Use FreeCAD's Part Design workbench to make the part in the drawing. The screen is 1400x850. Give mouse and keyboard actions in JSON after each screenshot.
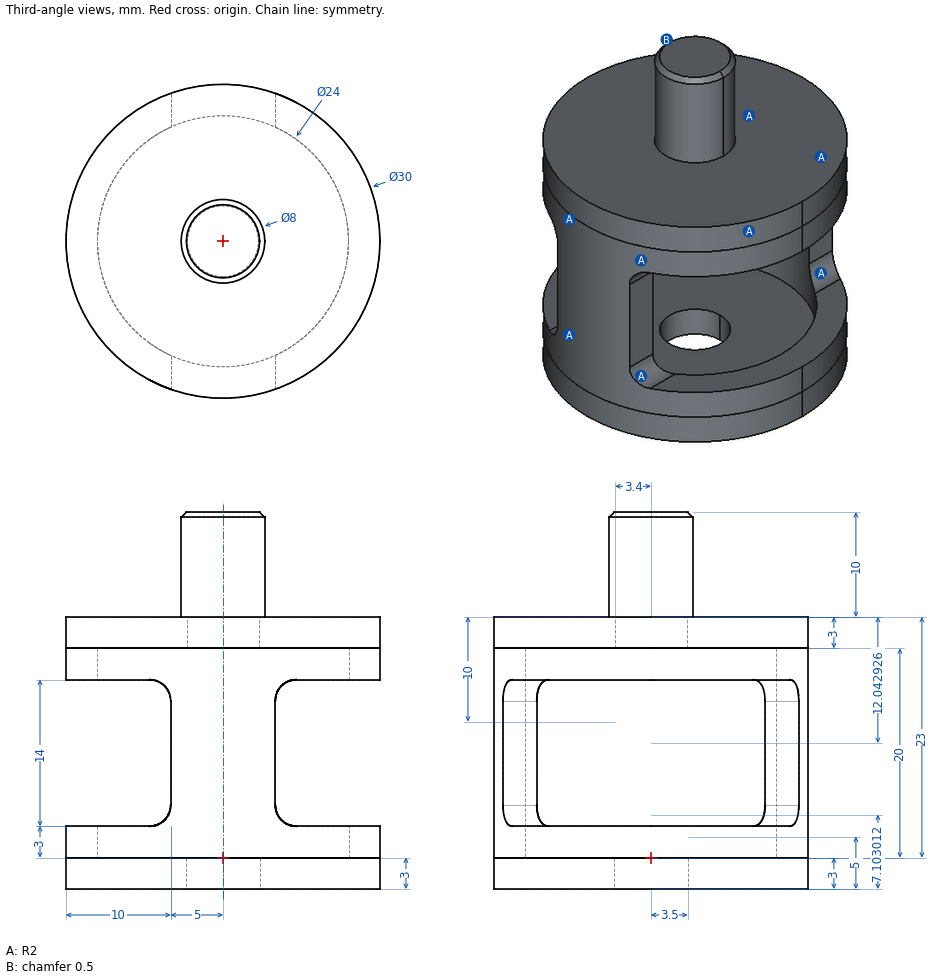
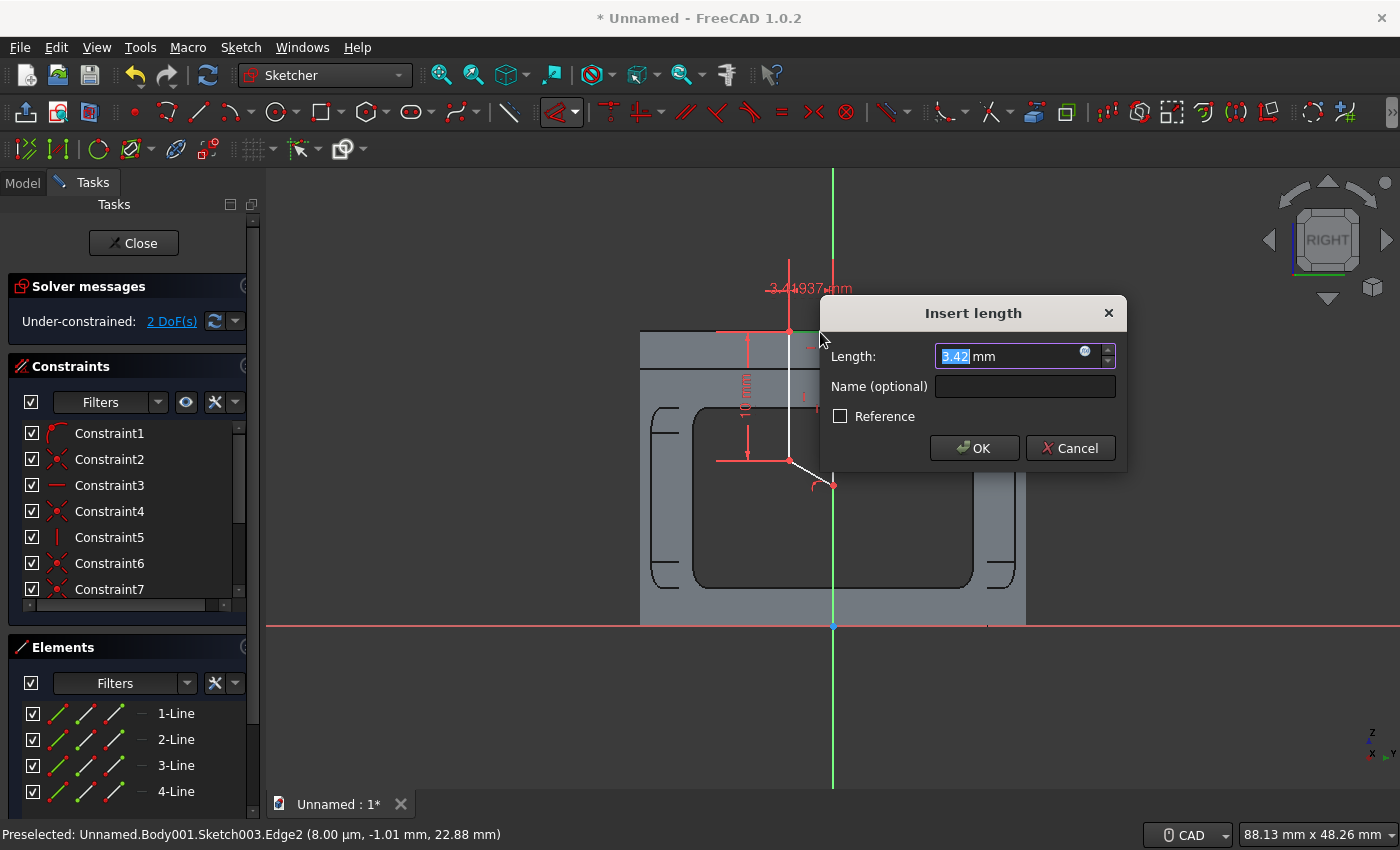
{"action": "type", "text": "3.4"}
{"action": "key", "text": "Return"}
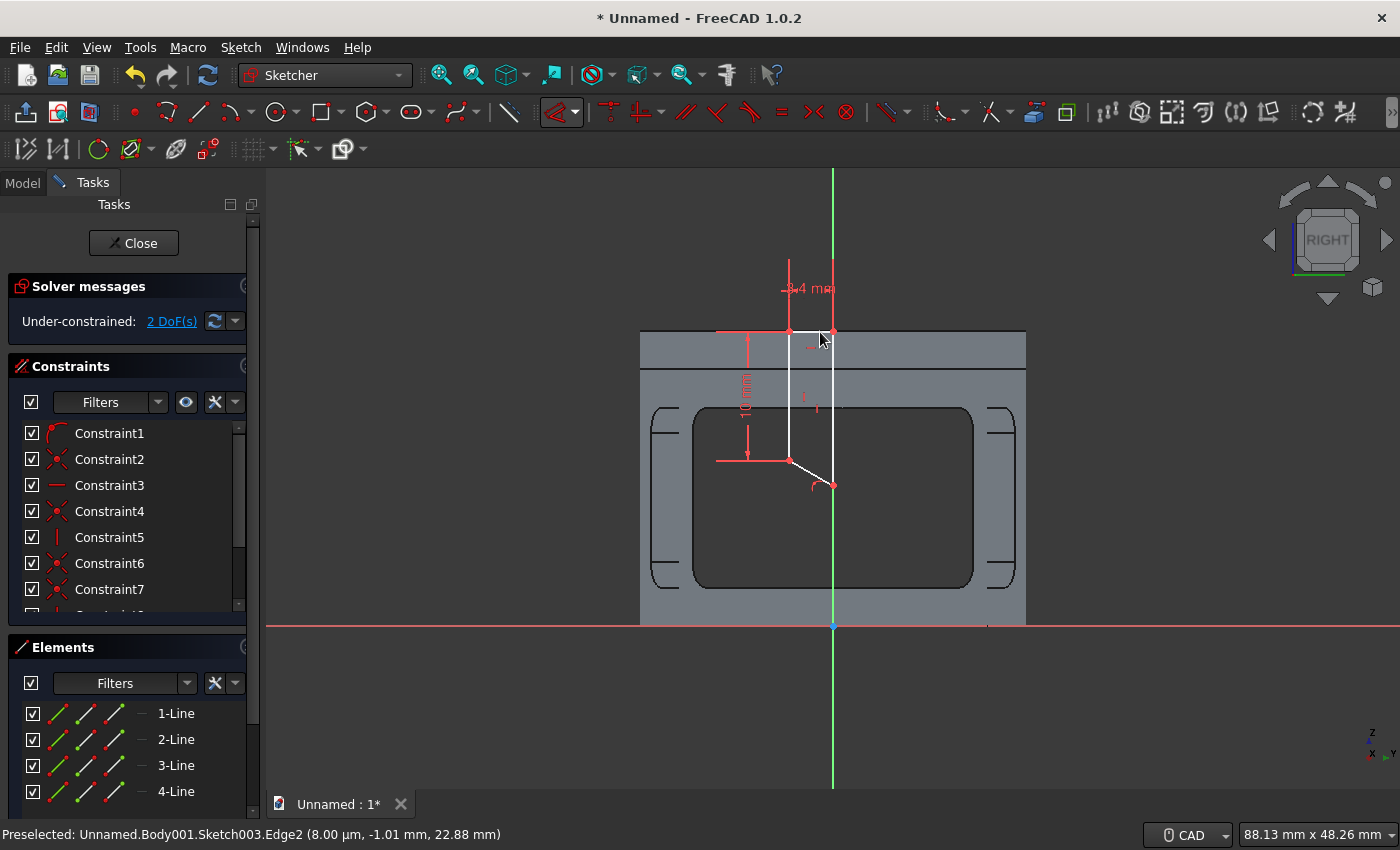
{"action": "left_click", "coordinate": [833, 332]}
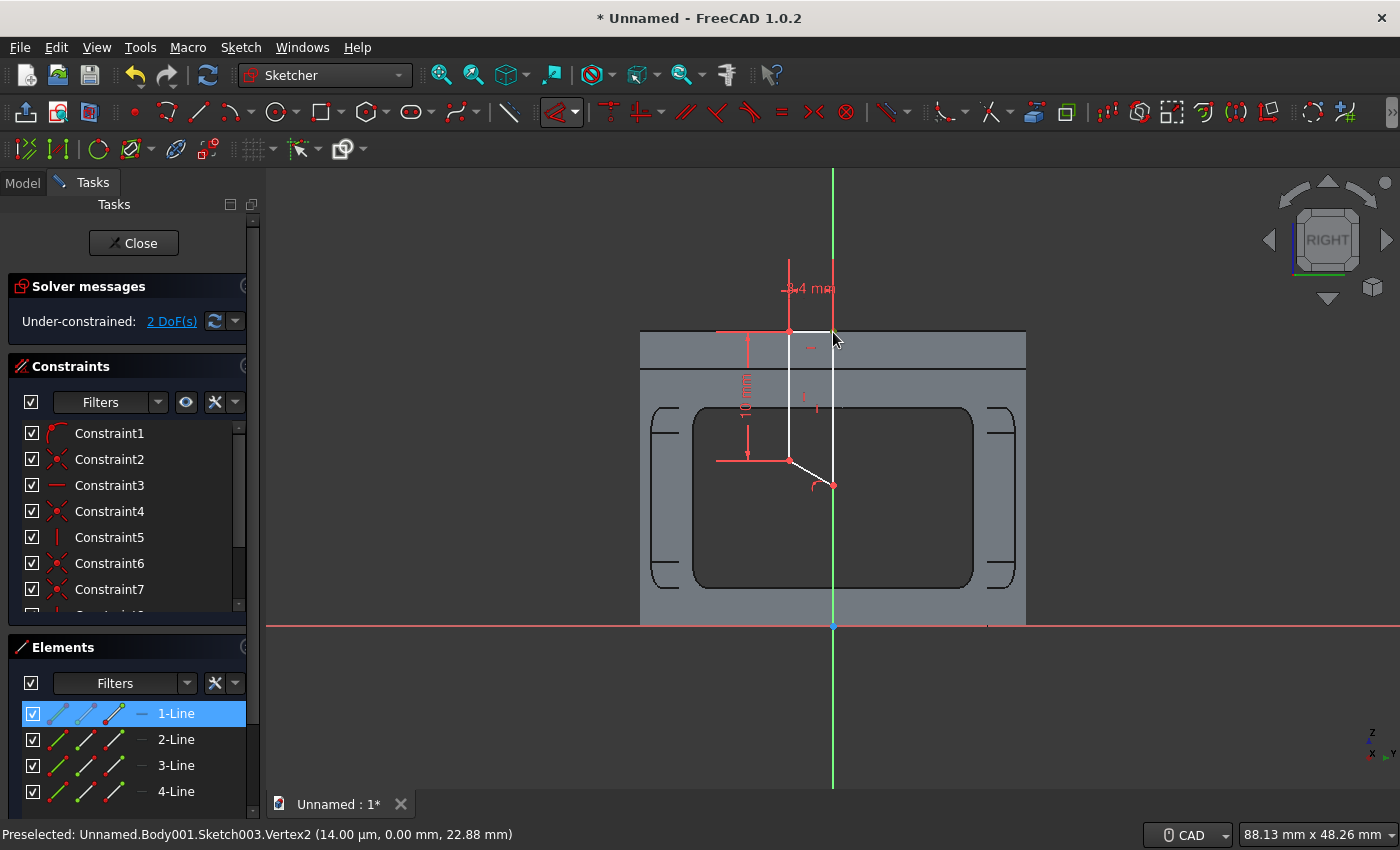
{"action": "key", "text": "i"}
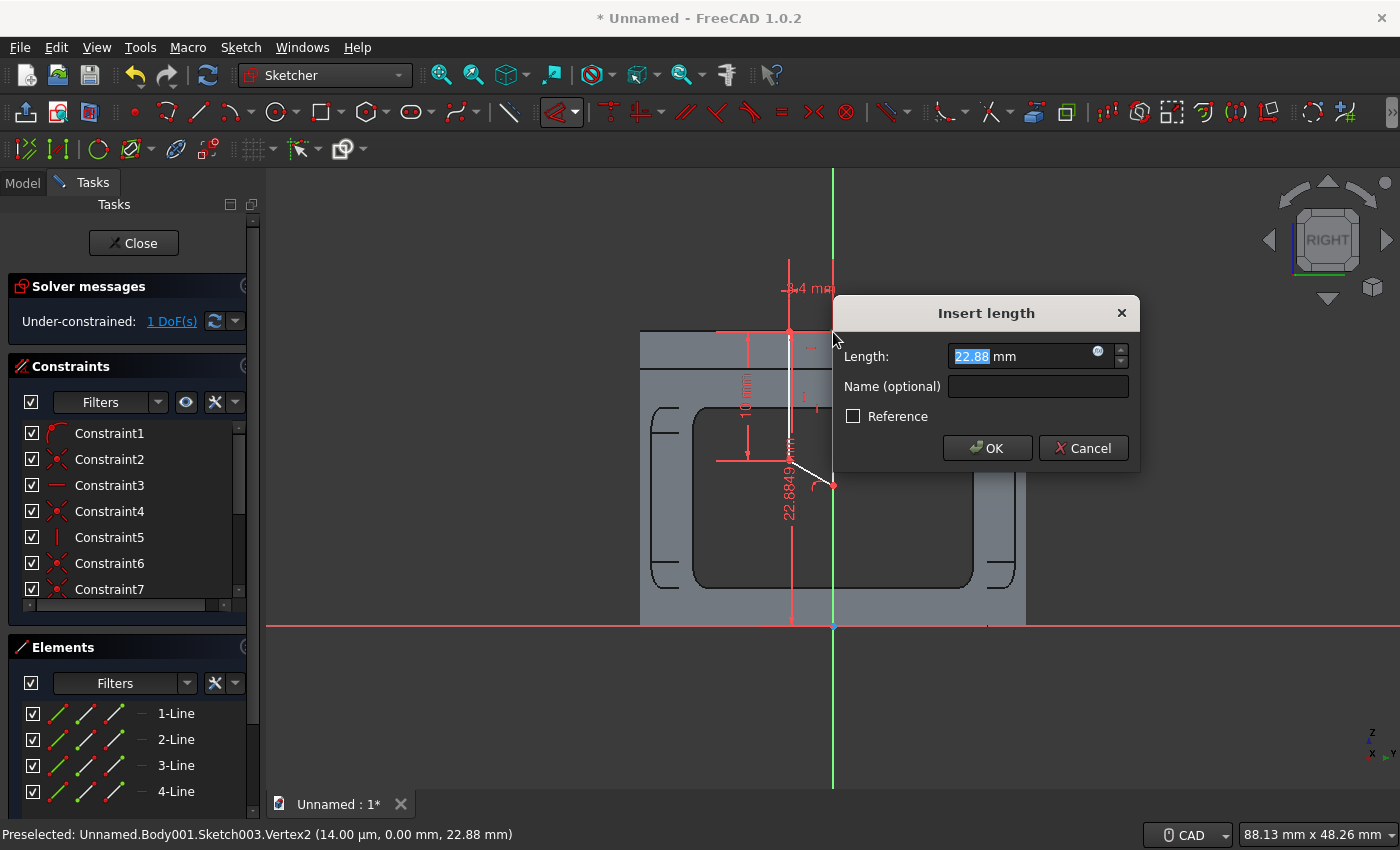
{"action": "type", "text": "23"}
{"action": "key", "text": "Return"}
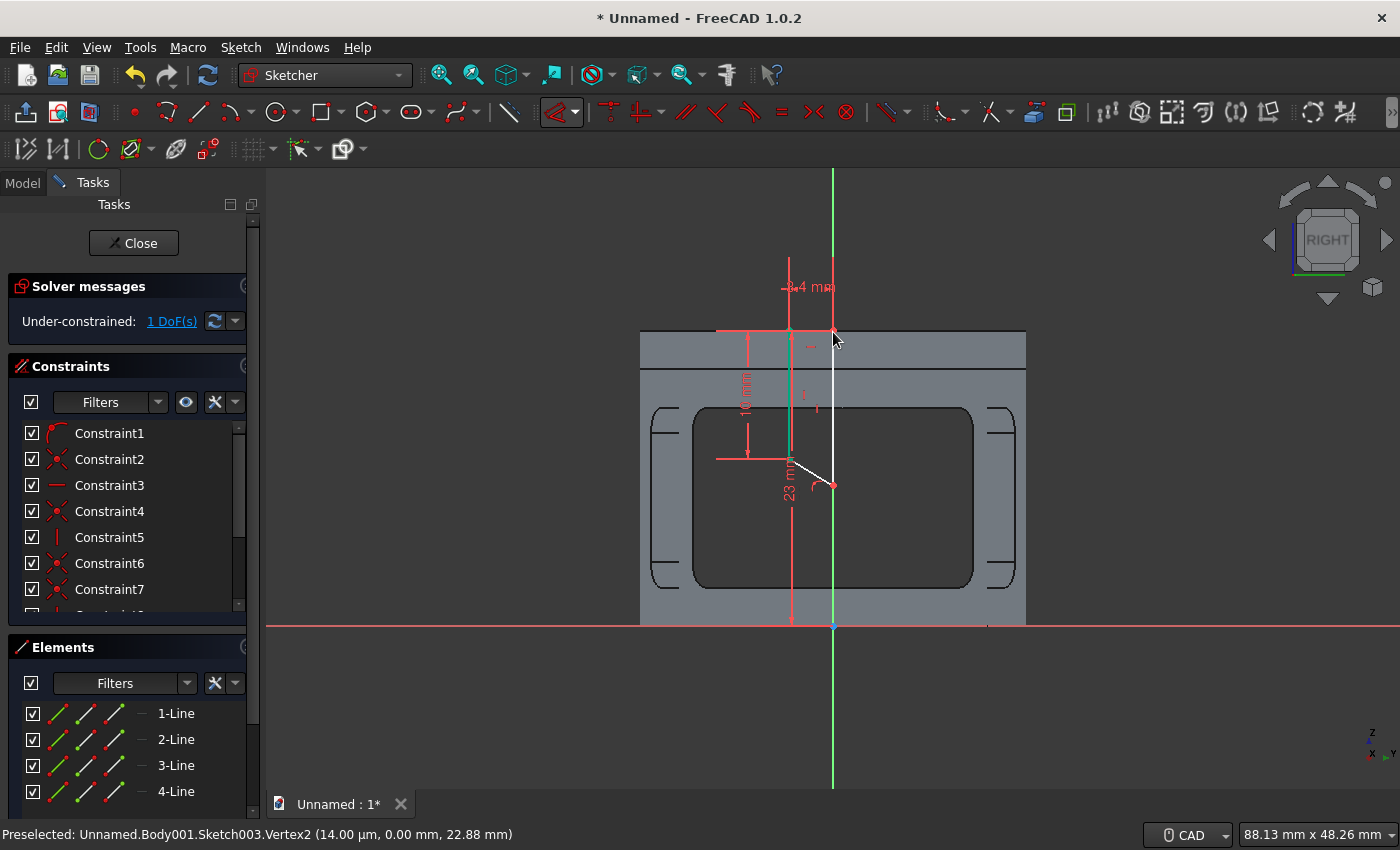
{"action": "left_click", "coordinate": [833, 439]}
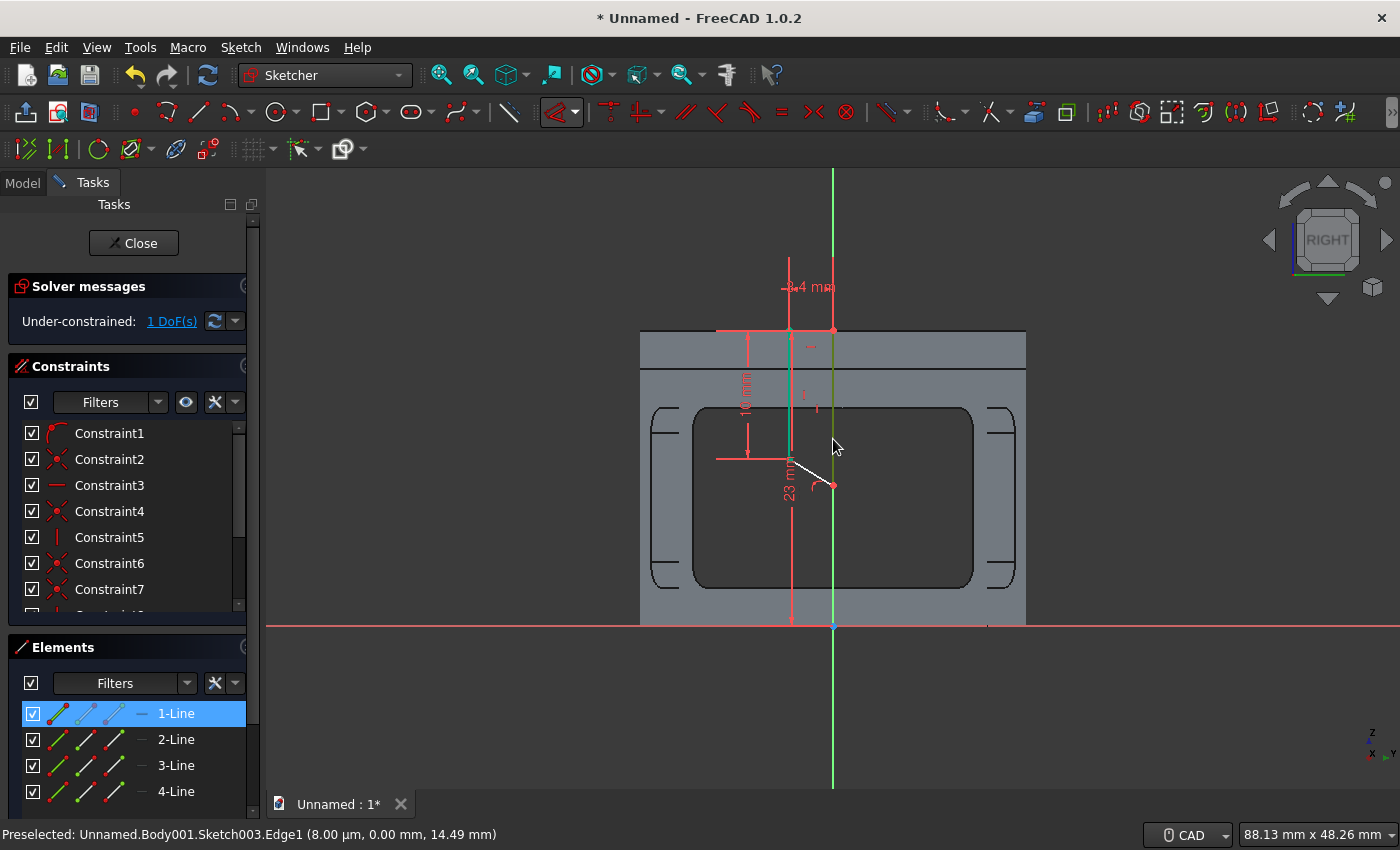
{"action": "key", "text": "i"}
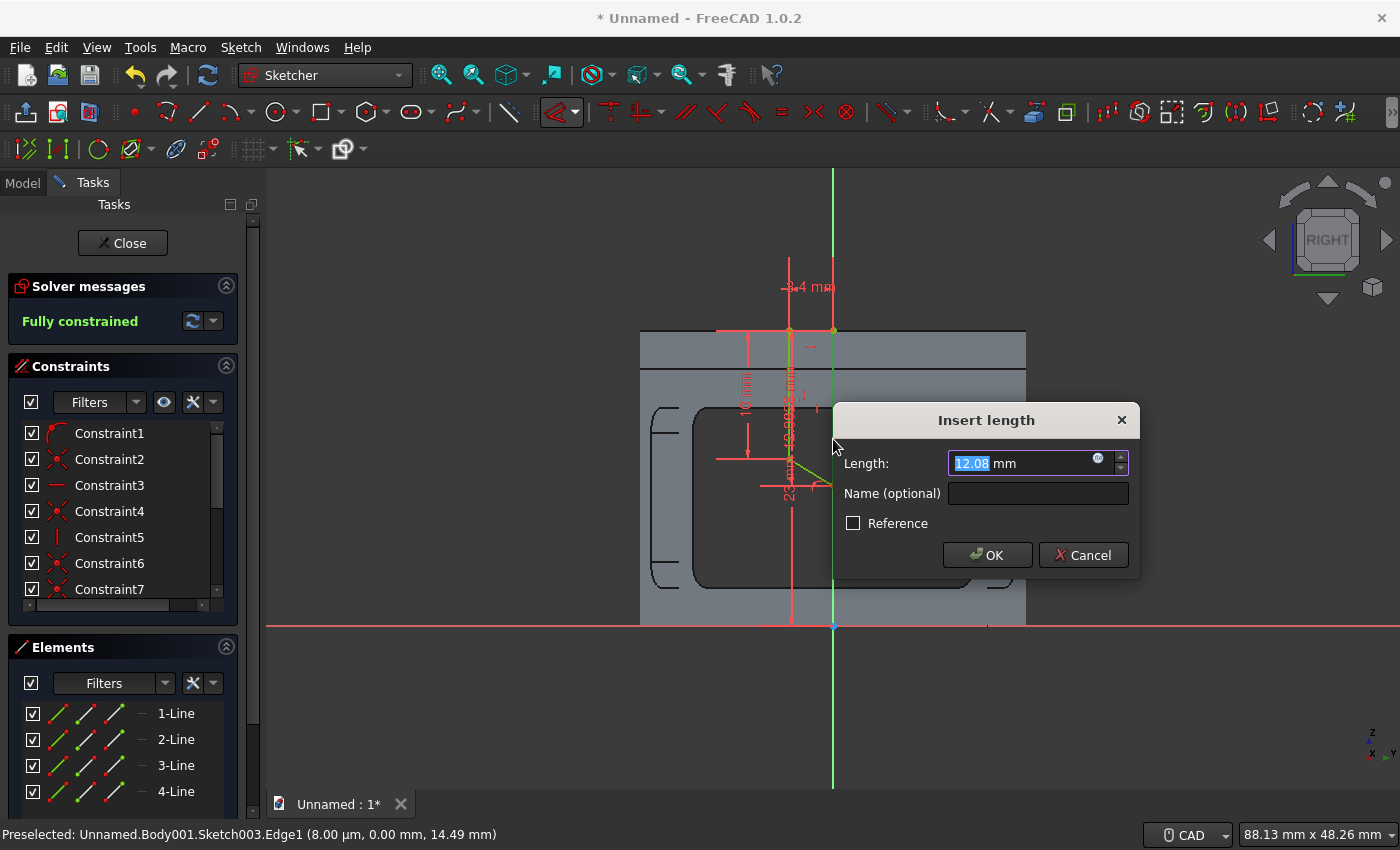
{"action": "type", "text": "12.042926"}
{"action": "key", "text": "Return"}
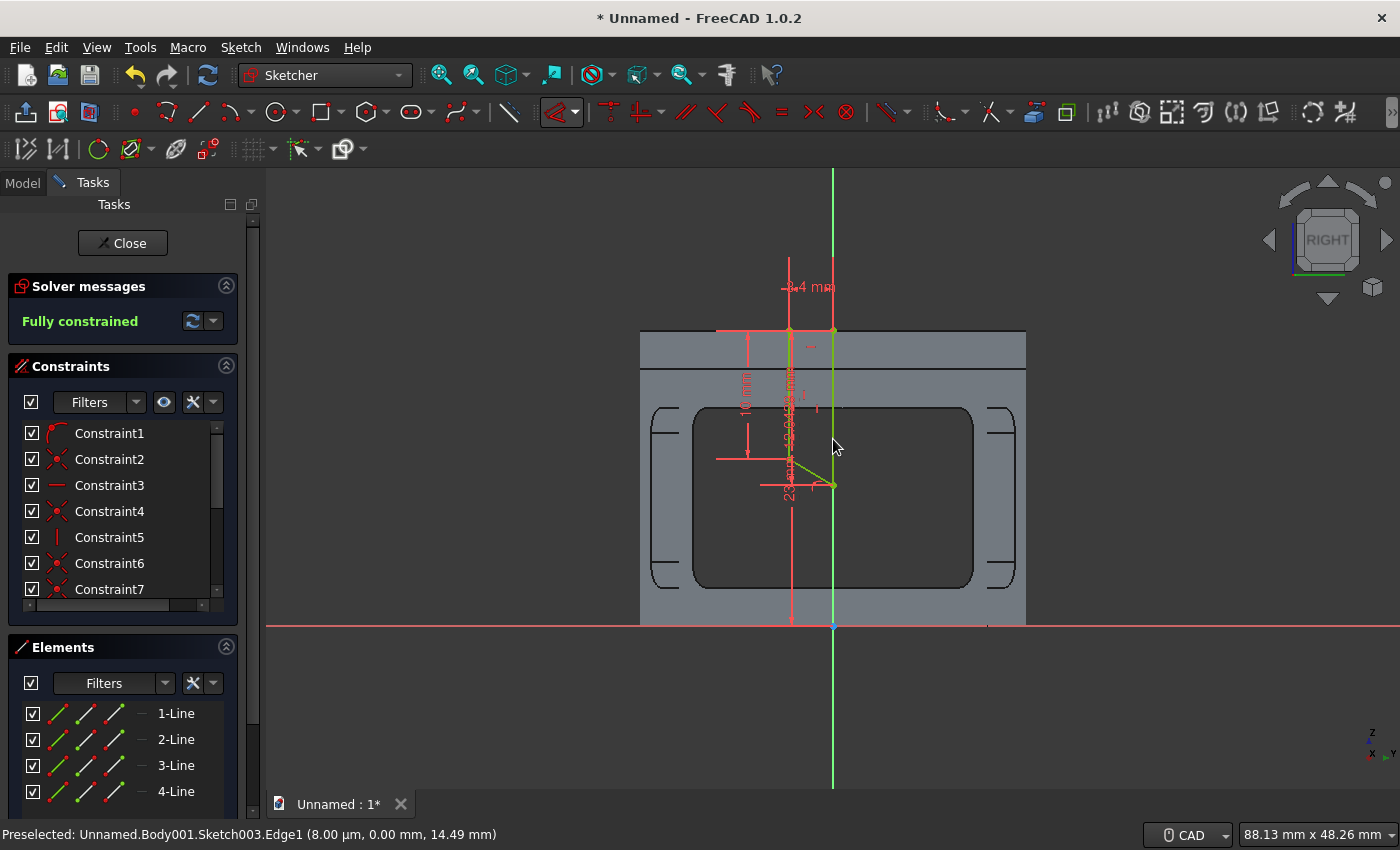
{"action": "left_click", "coordinate": [123, 243]}